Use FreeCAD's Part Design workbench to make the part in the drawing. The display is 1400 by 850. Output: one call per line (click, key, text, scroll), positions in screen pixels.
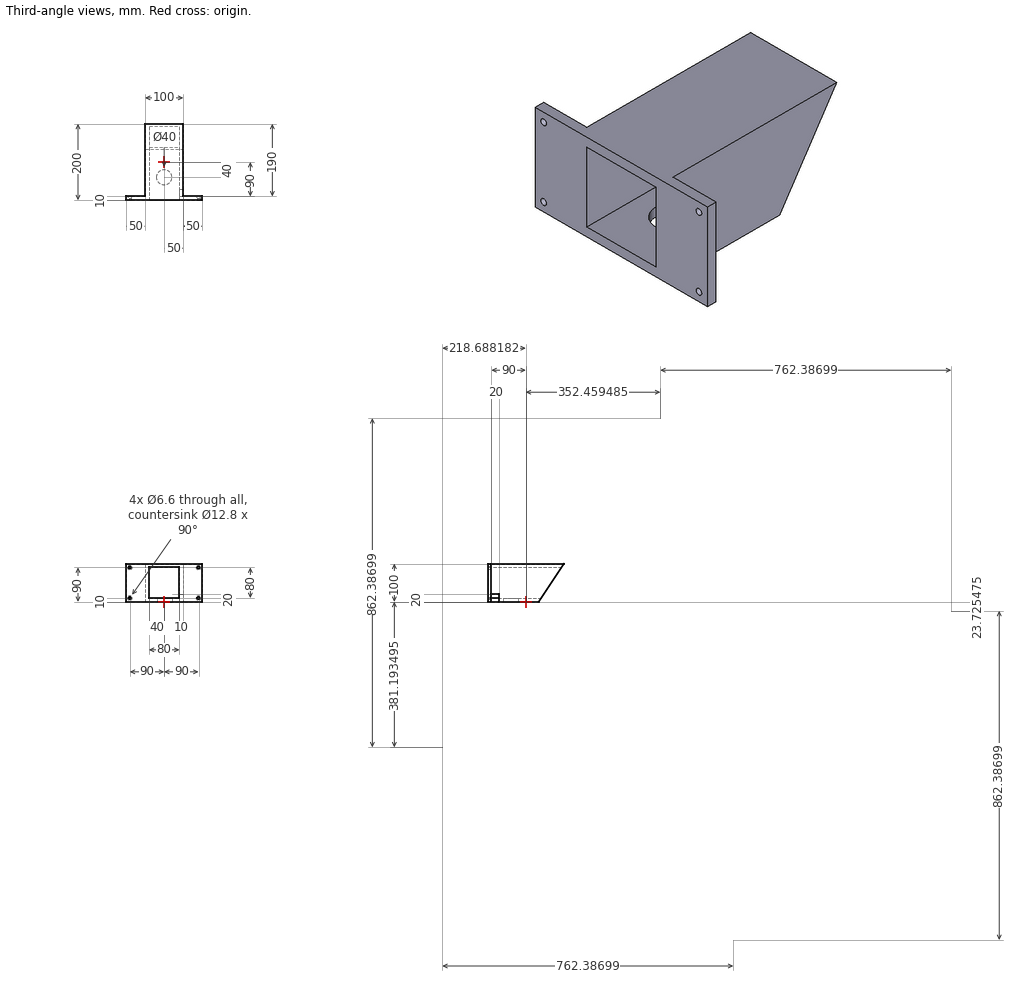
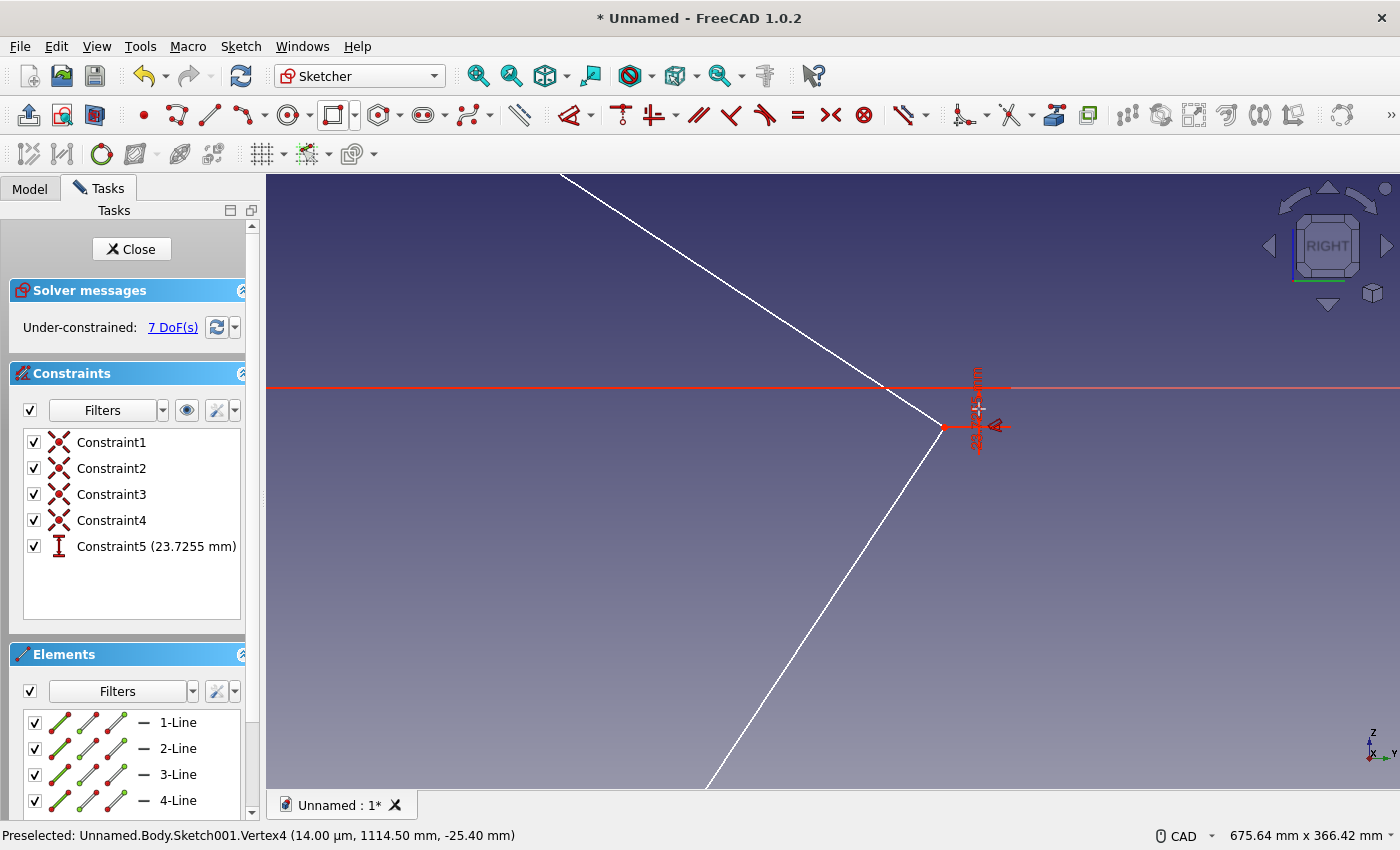
scroll(950, 433, down, 9)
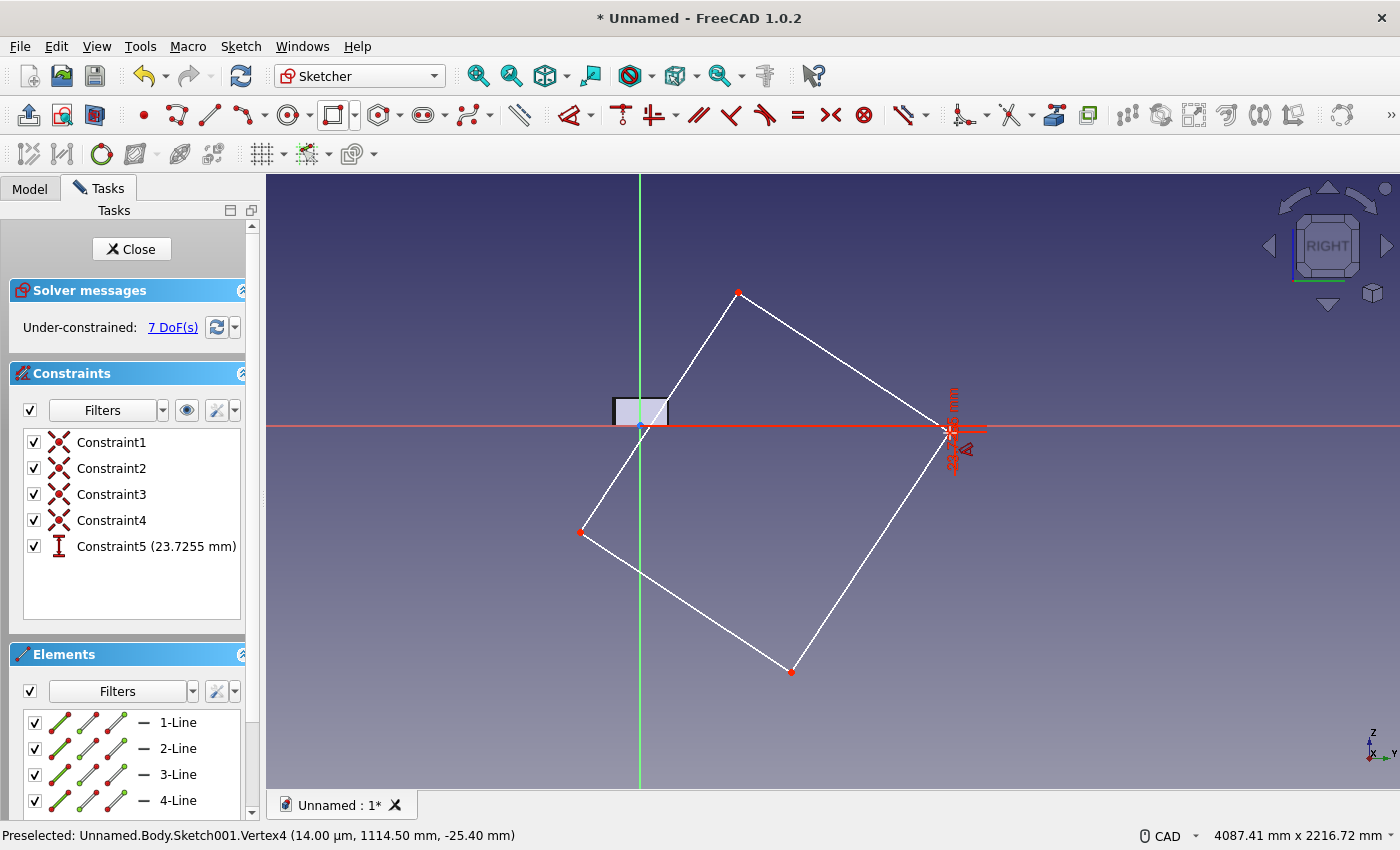
scroll(643, 575, up, 8)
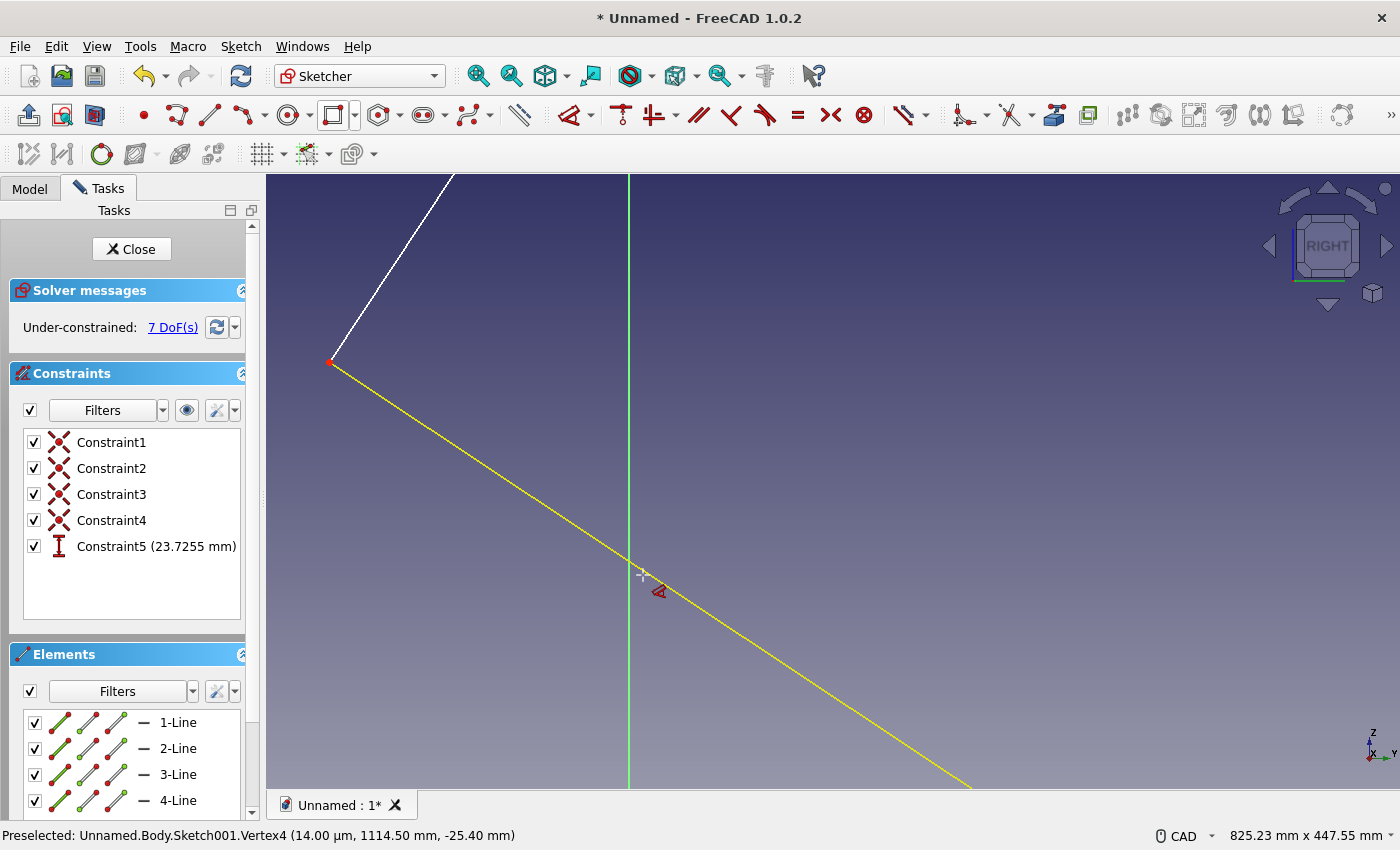
click(643, 571)
click(782, 329)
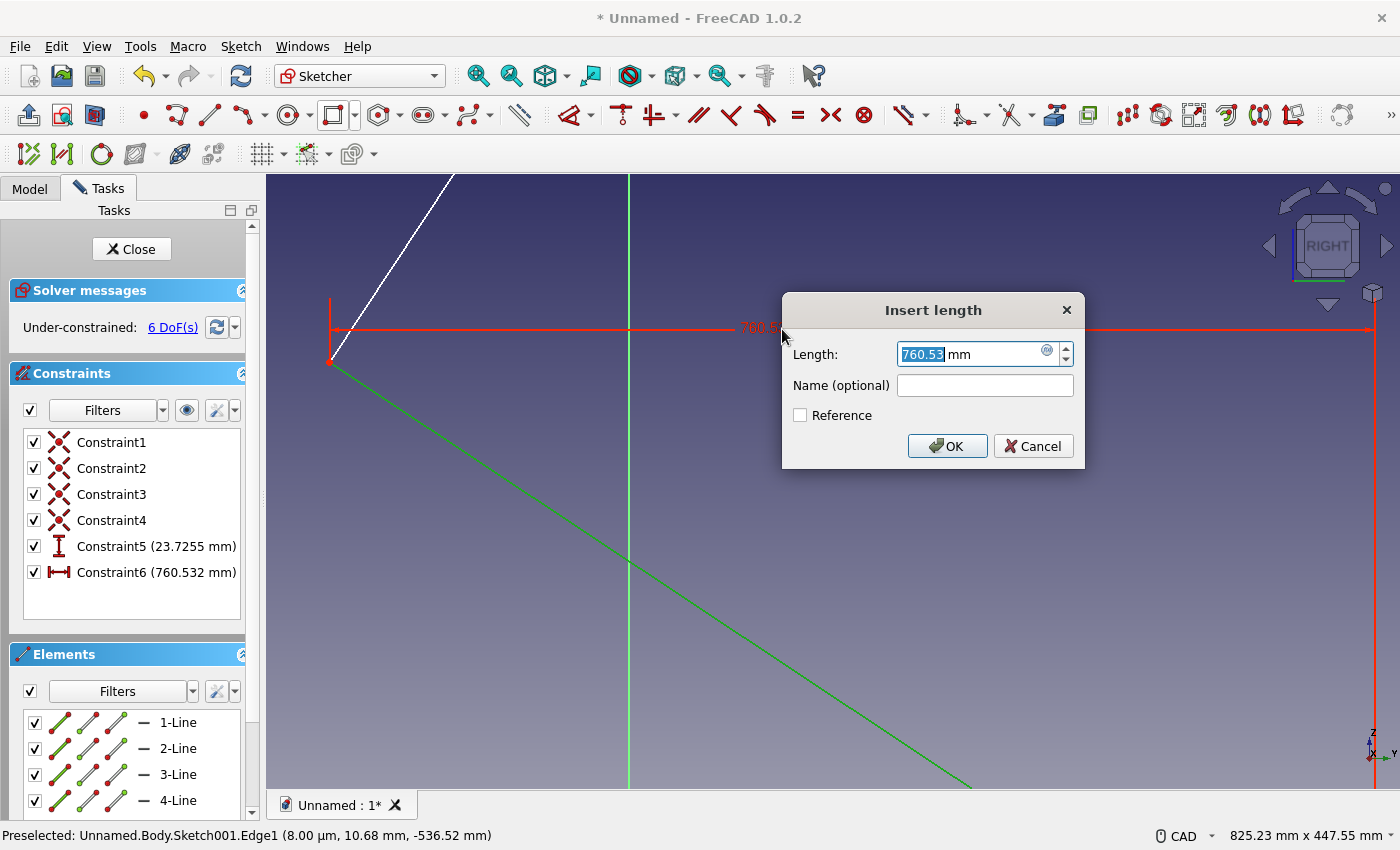
text(762.38699)
key(Return)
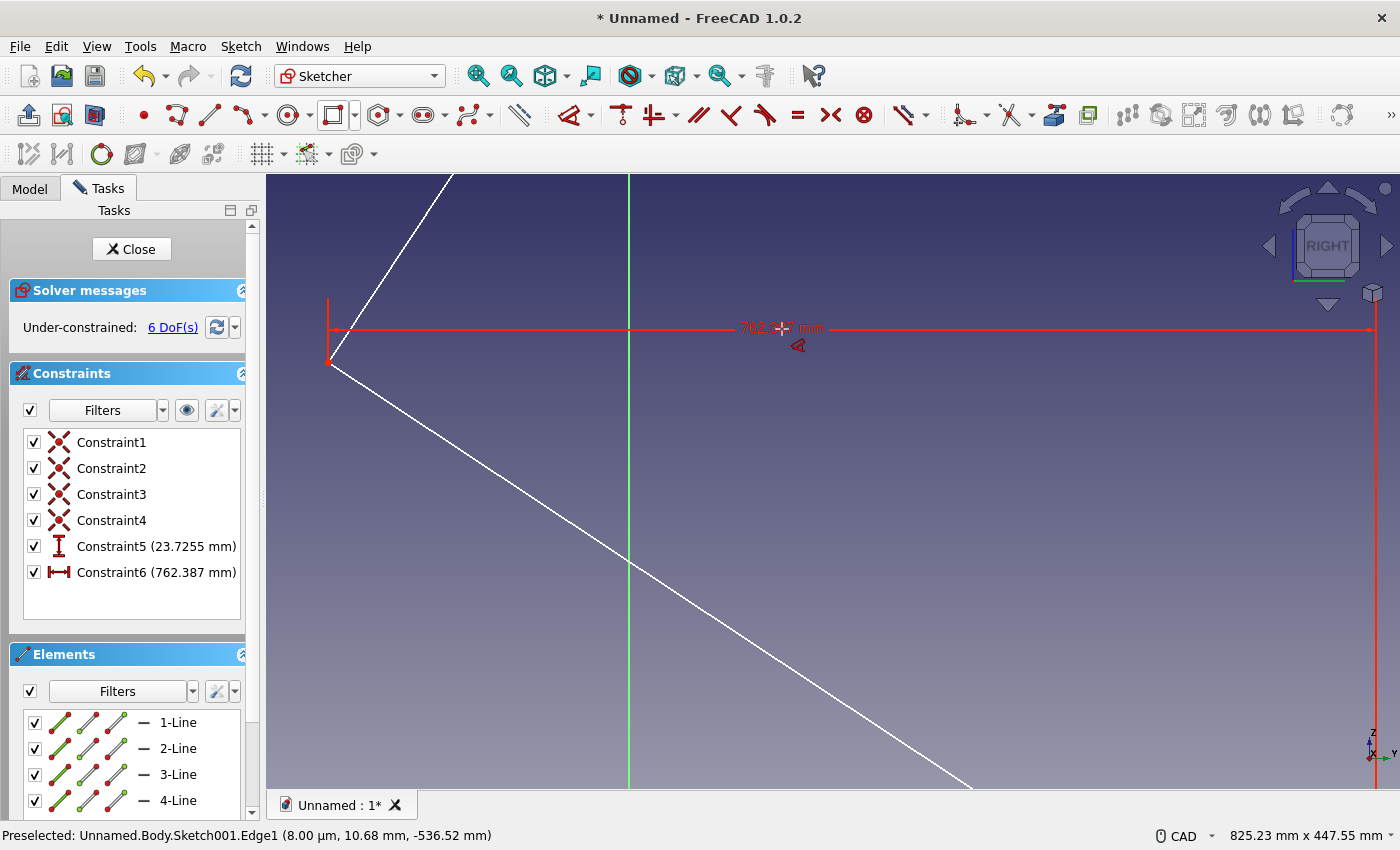
scroll(643, 575, down, 8)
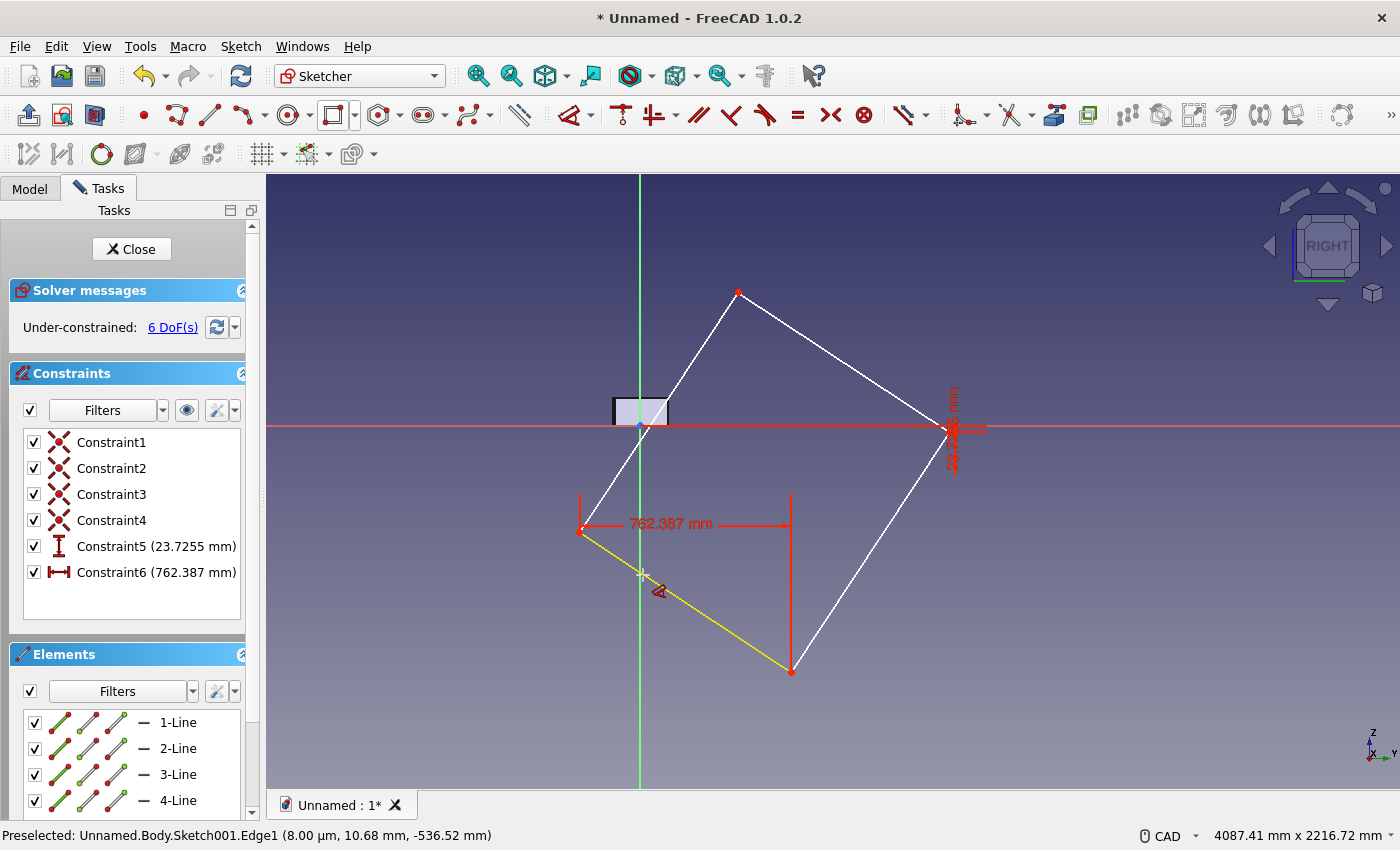
click(839, 601)
click(984, 553)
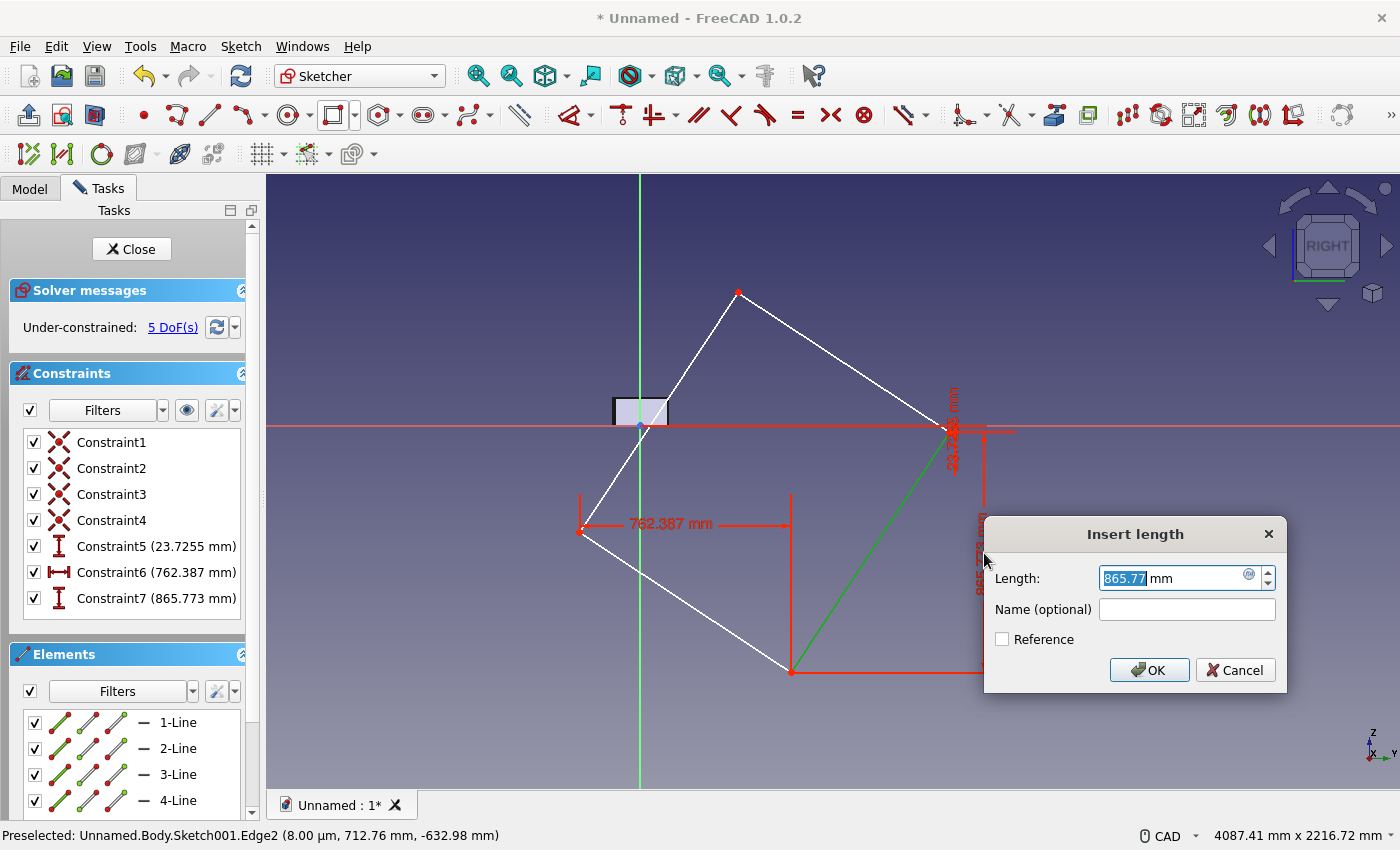
text(862.38699)
key(Return)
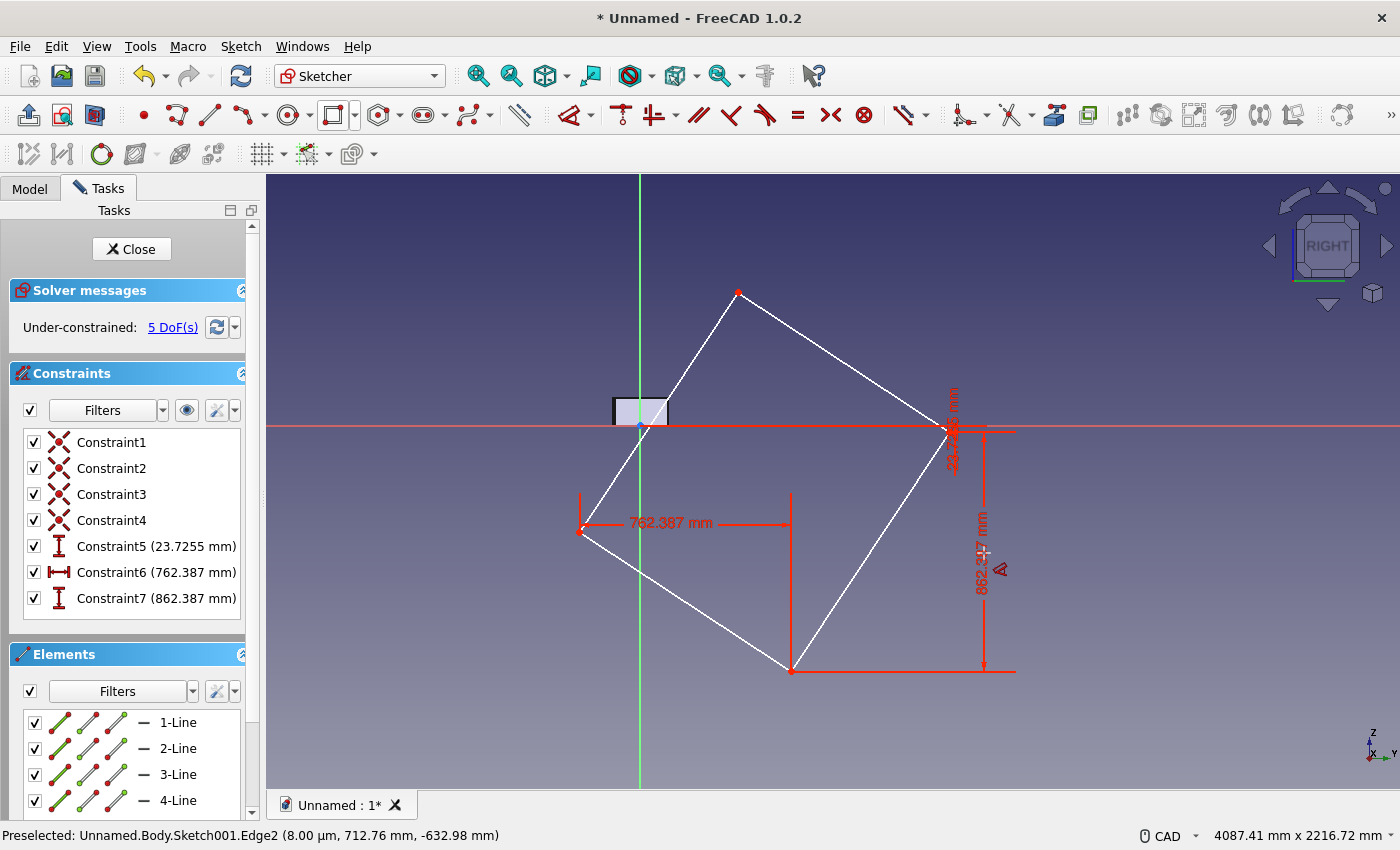
click(886, 391)
click(844, 259)